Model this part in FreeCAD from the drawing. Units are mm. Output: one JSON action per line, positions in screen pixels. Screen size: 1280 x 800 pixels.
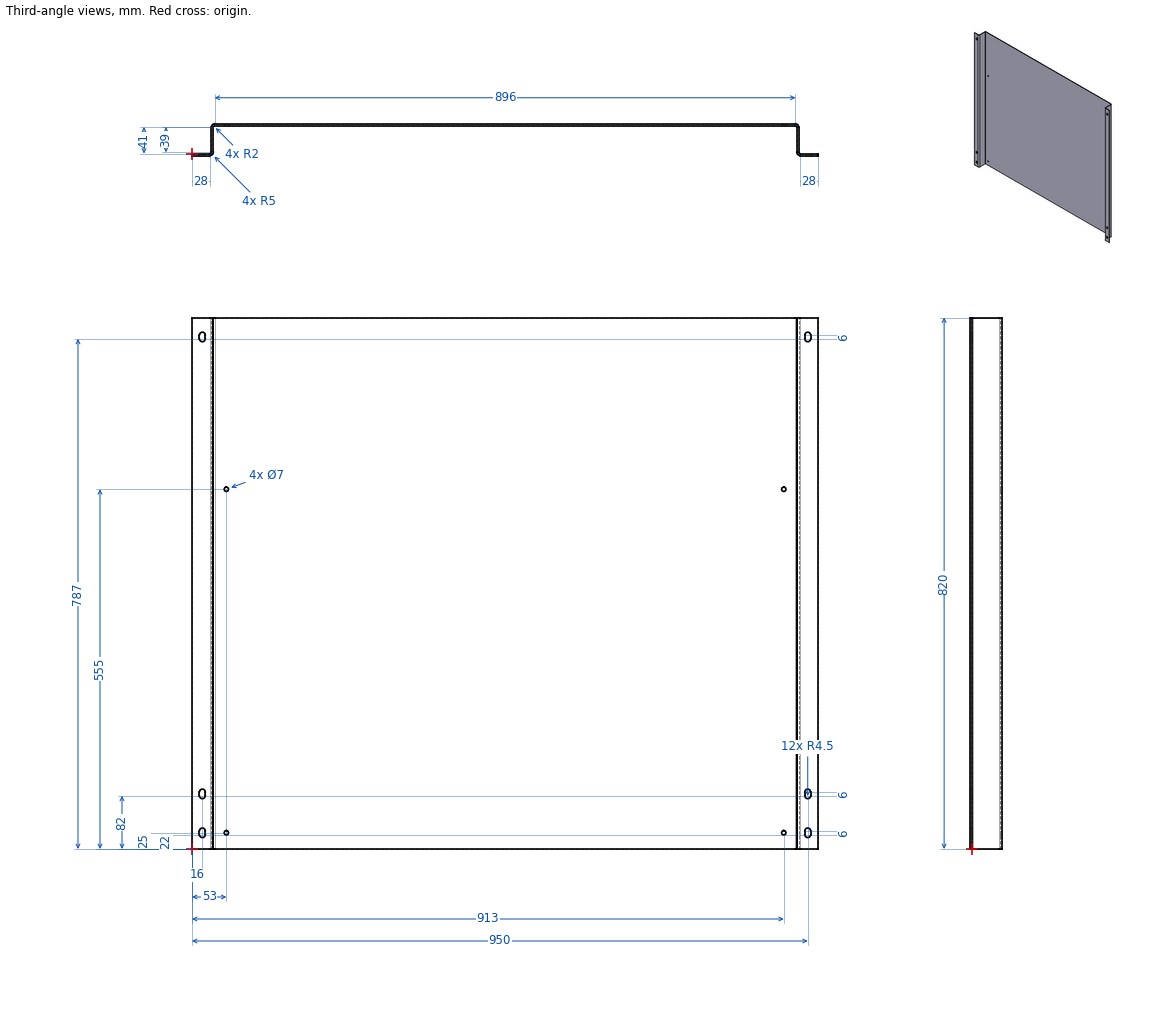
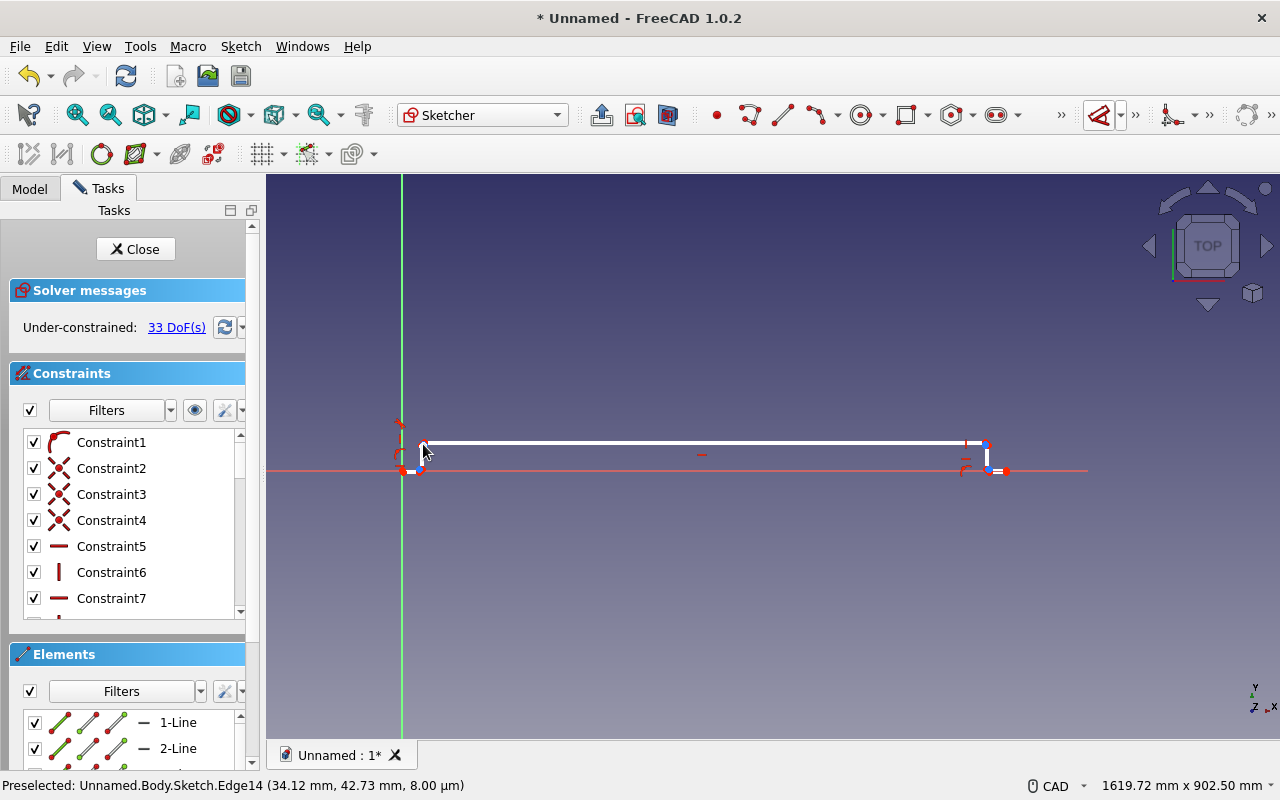
{"action": "scroll", "coordinate": [592, 444], "scroll_direction": "up", "scroll_amount": 10}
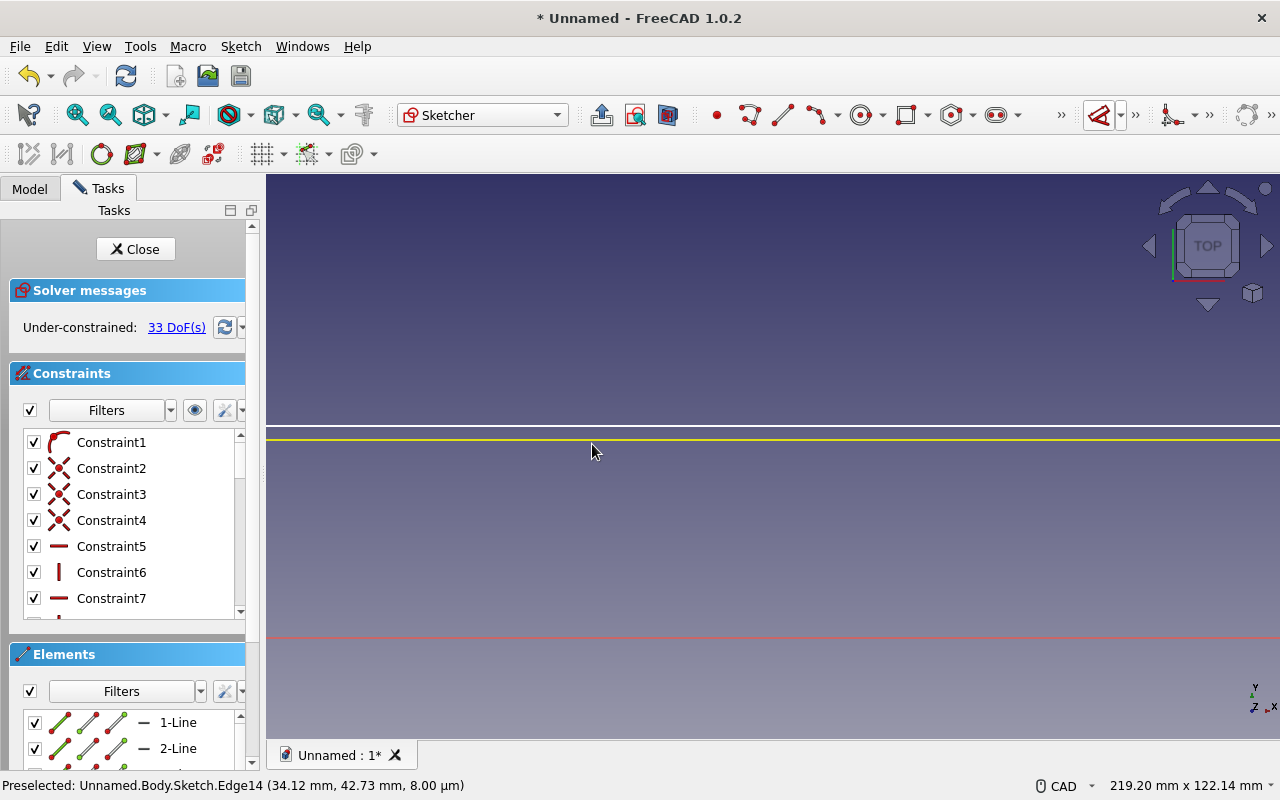
{"action": "left_click", "coordinate": [593, 440]}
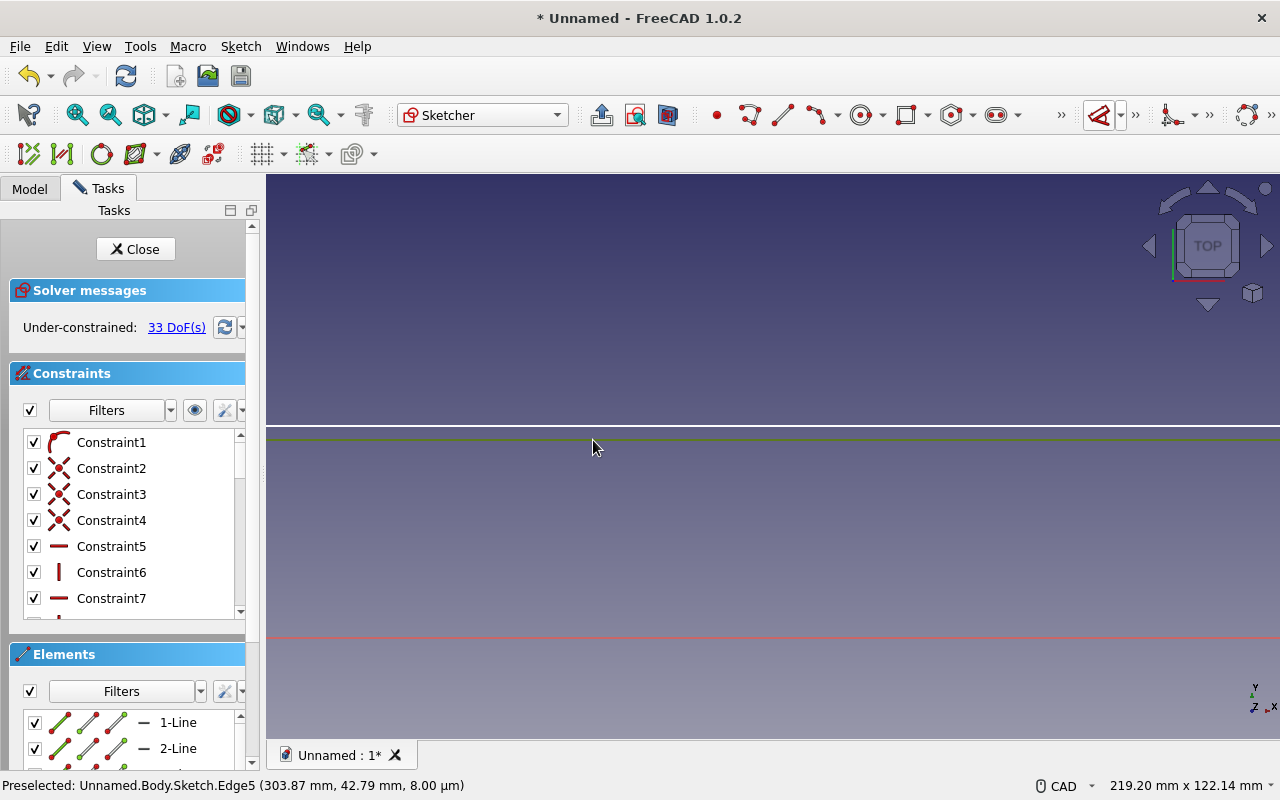
{"action": "scroll", "coordinate": [592, 444], "scroll_direction": "down", "scroll_amount": 10}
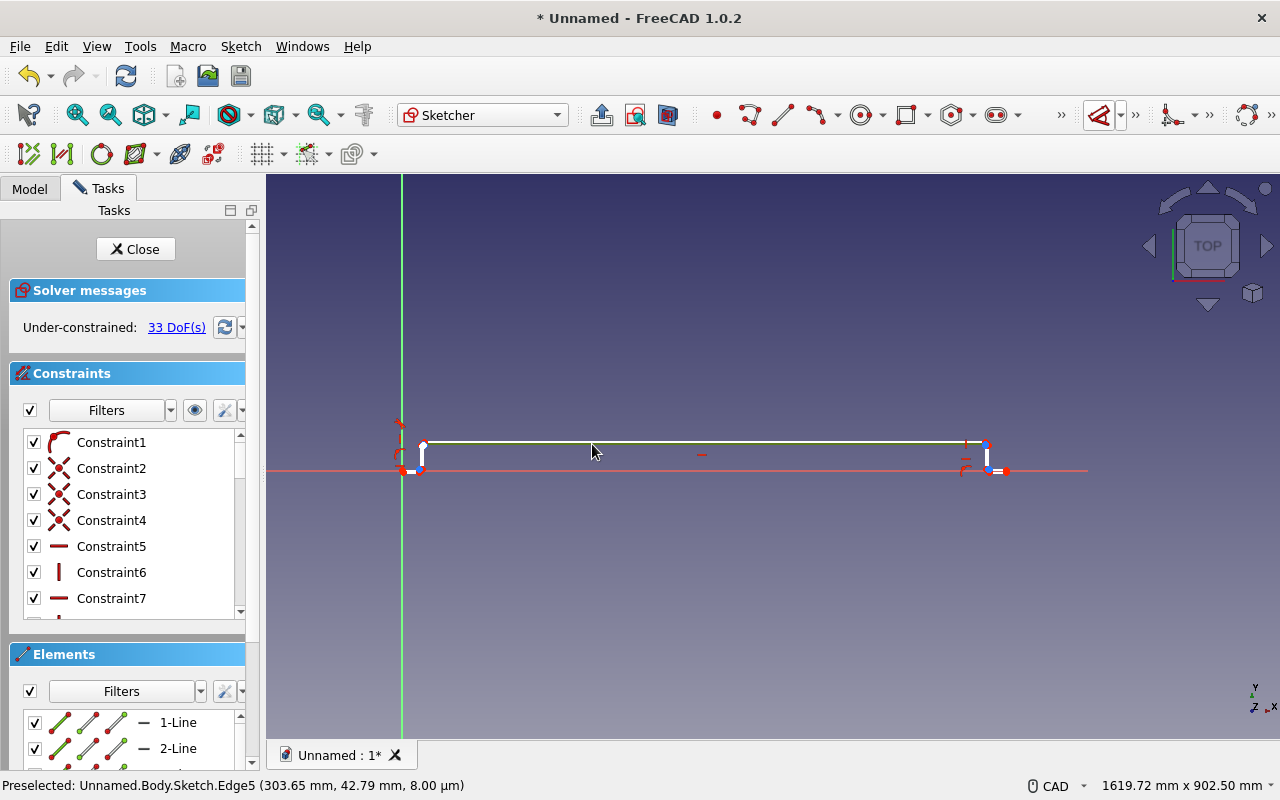
{"action": "scroll", "coordinate": [423, 444], "scroll_direction": "up", "scroll_amount": 14}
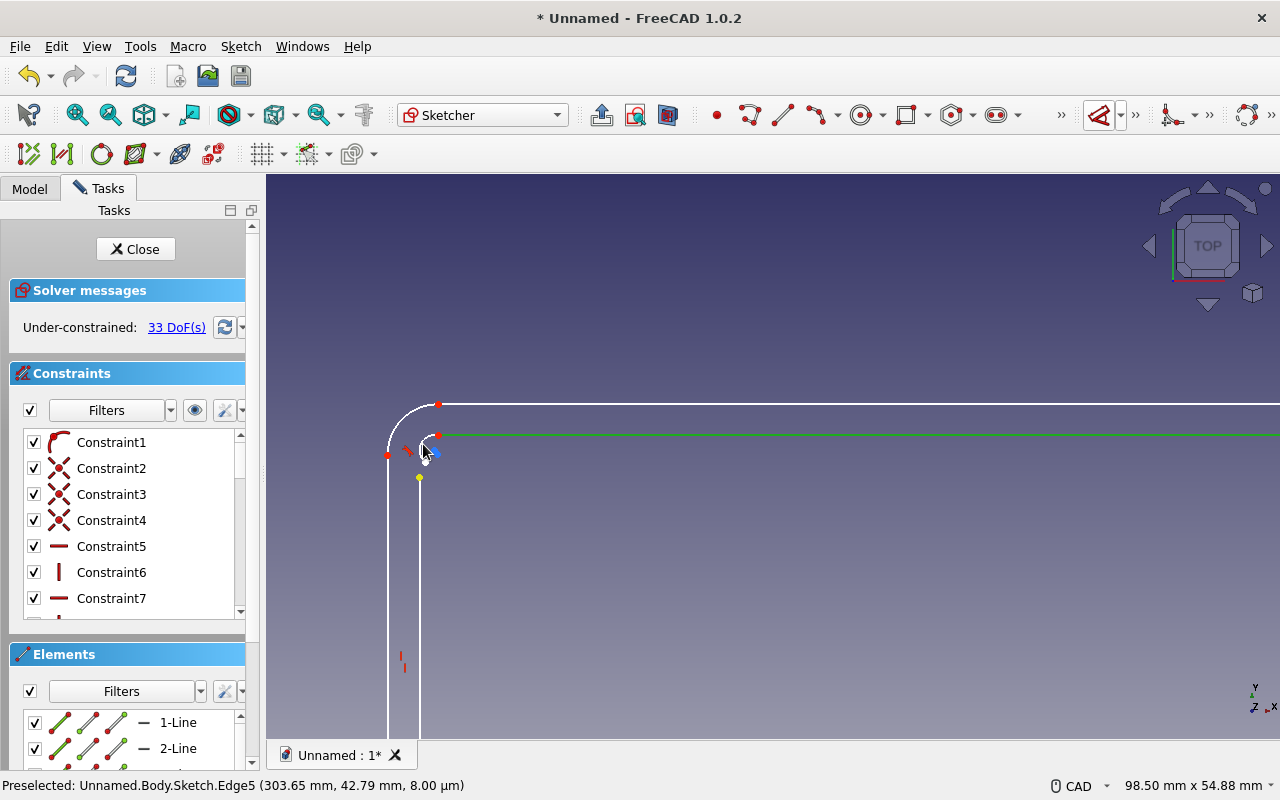
{"action": "left_click", "coordinate": [421, 444]}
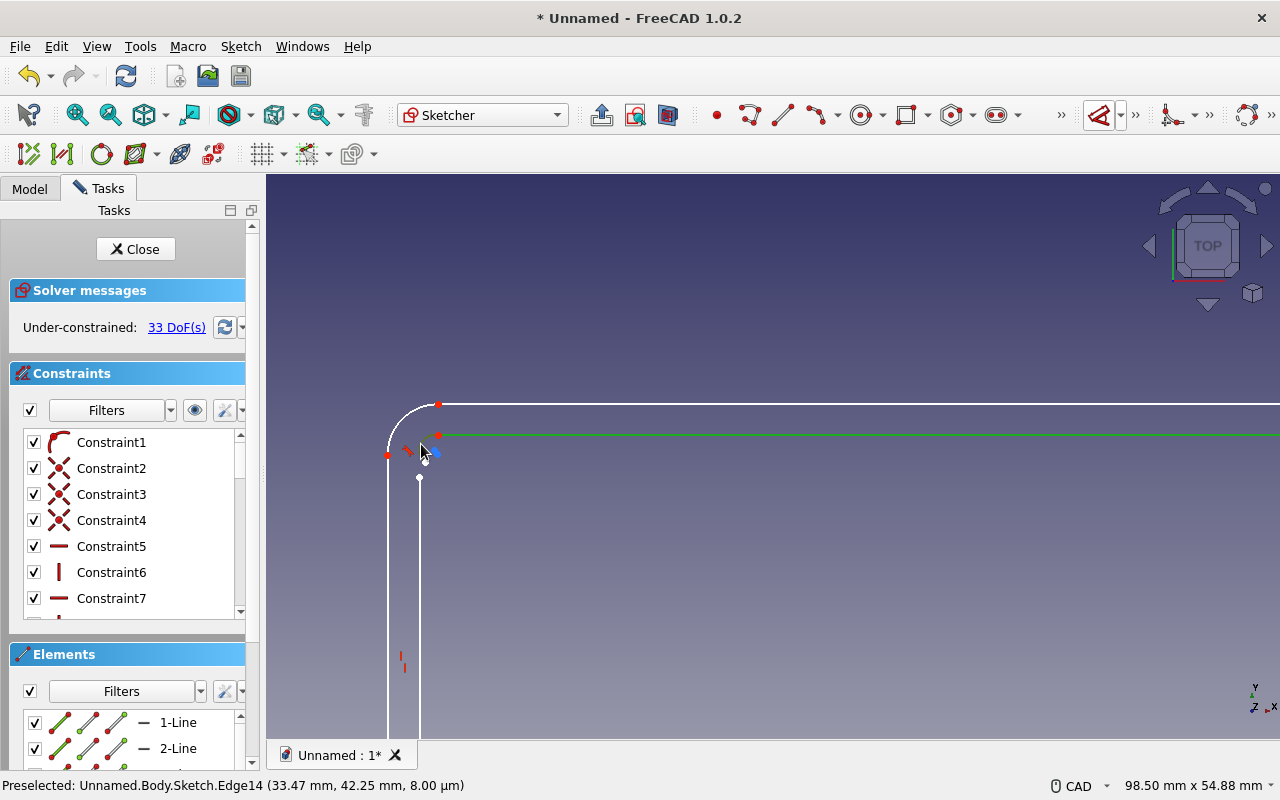
{"action": "key", "text": "t"}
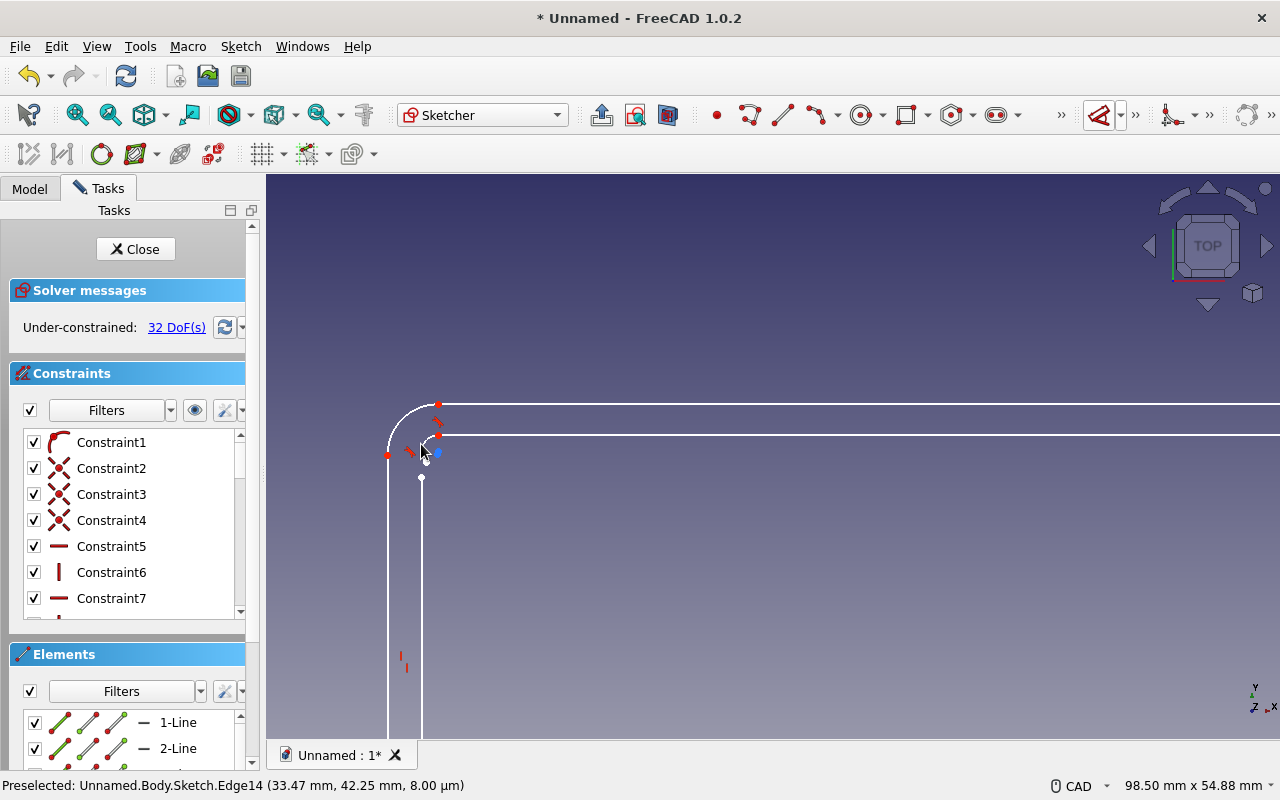
{"action": "scroll", "coordinate": [423, 444], "scroll_direction": "down", "scroll_amount": 14}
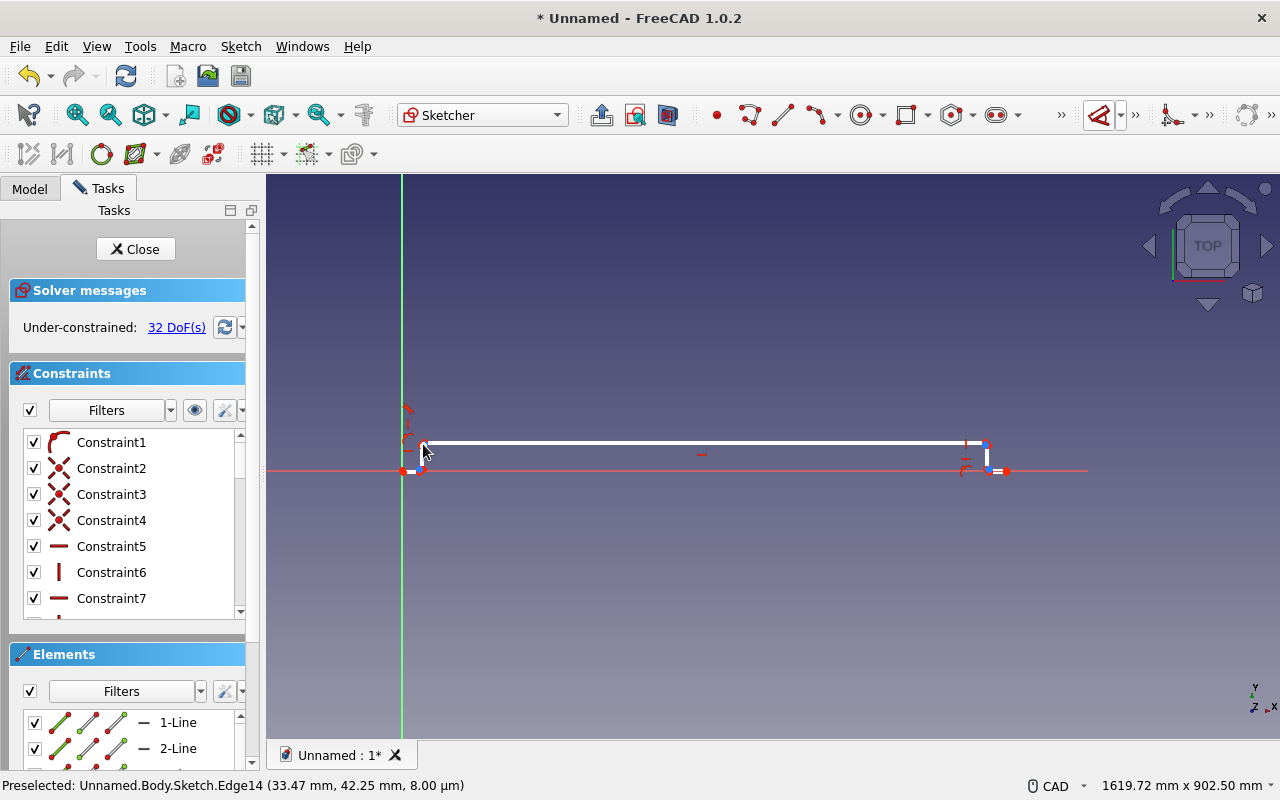
{"action": "scroll", "coordinate": [592, 444], "scroll_direction": "up", "scroll_amount": 10}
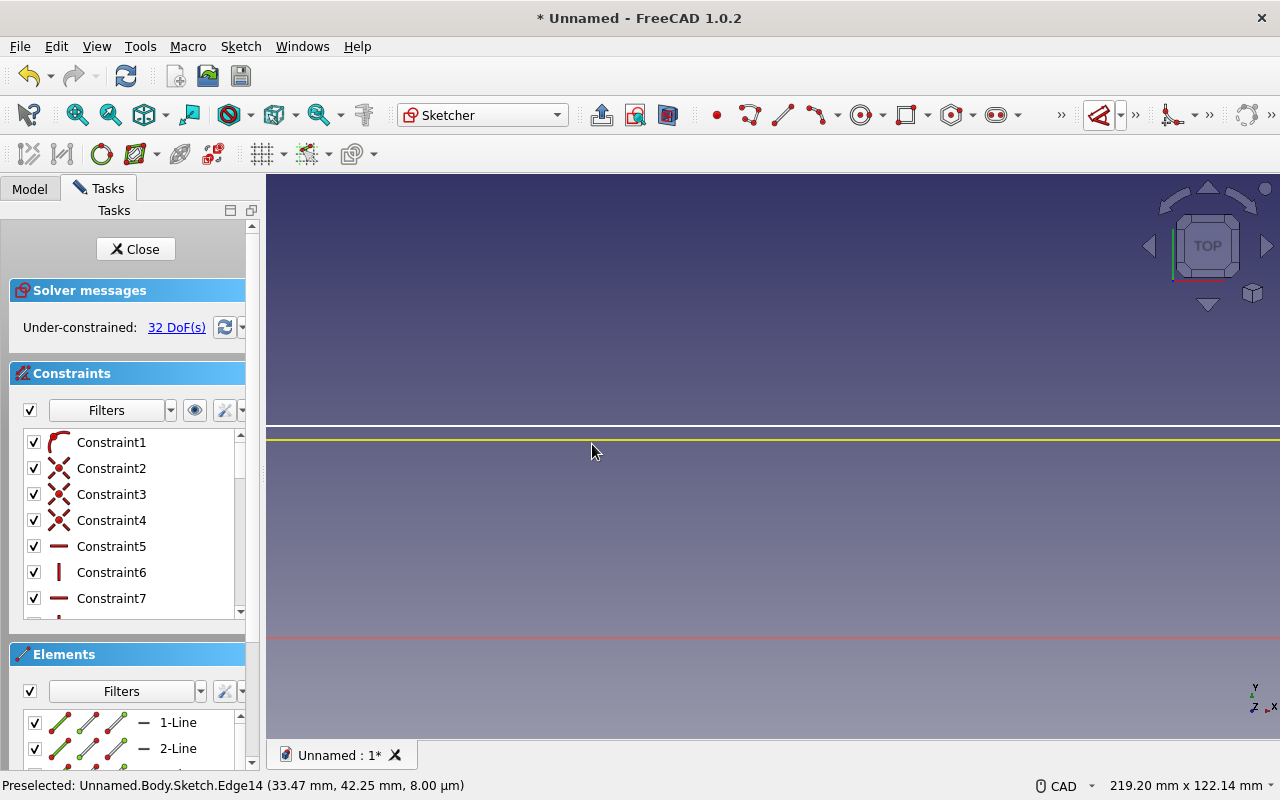
{"action": "left_click", "coordinate": [593, 440]}